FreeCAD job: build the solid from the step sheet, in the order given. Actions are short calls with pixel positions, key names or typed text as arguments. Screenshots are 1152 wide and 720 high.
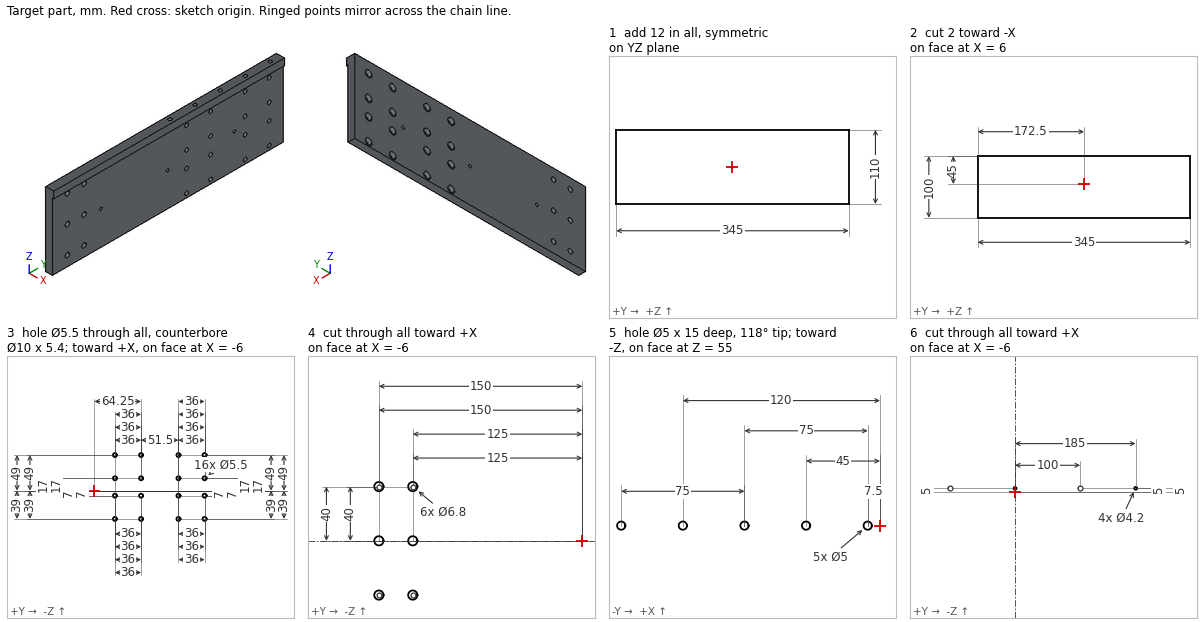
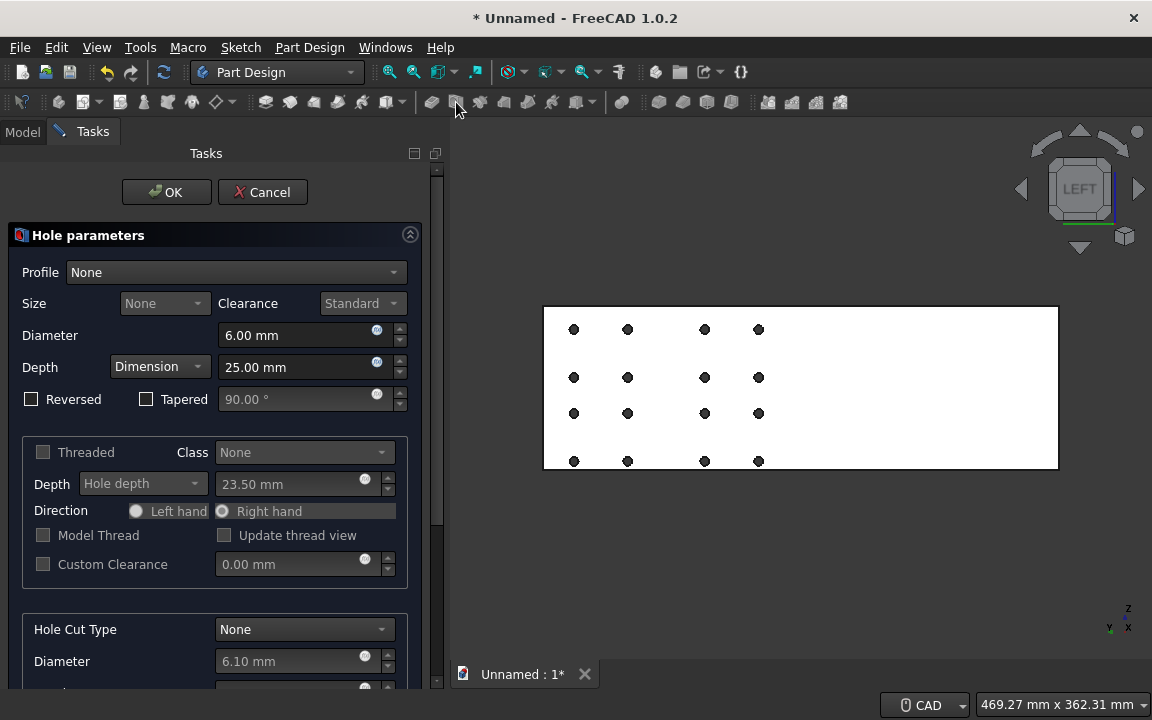
triple_click(305, 335)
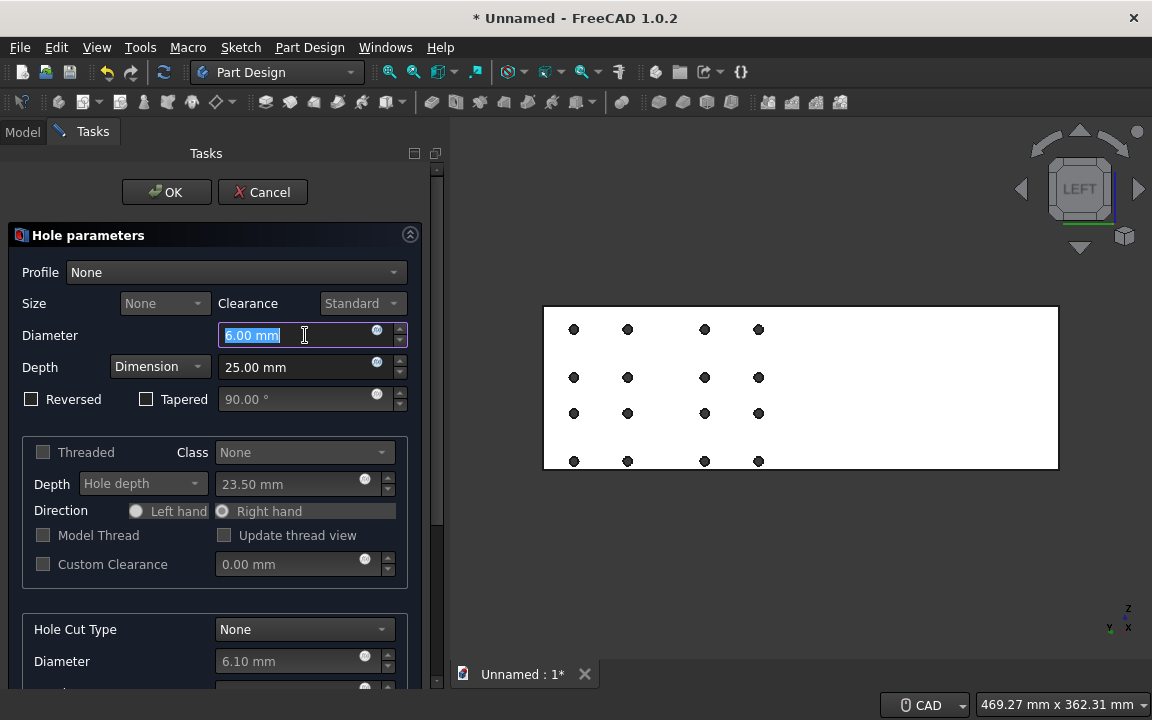
text(5.5)
key(Tab)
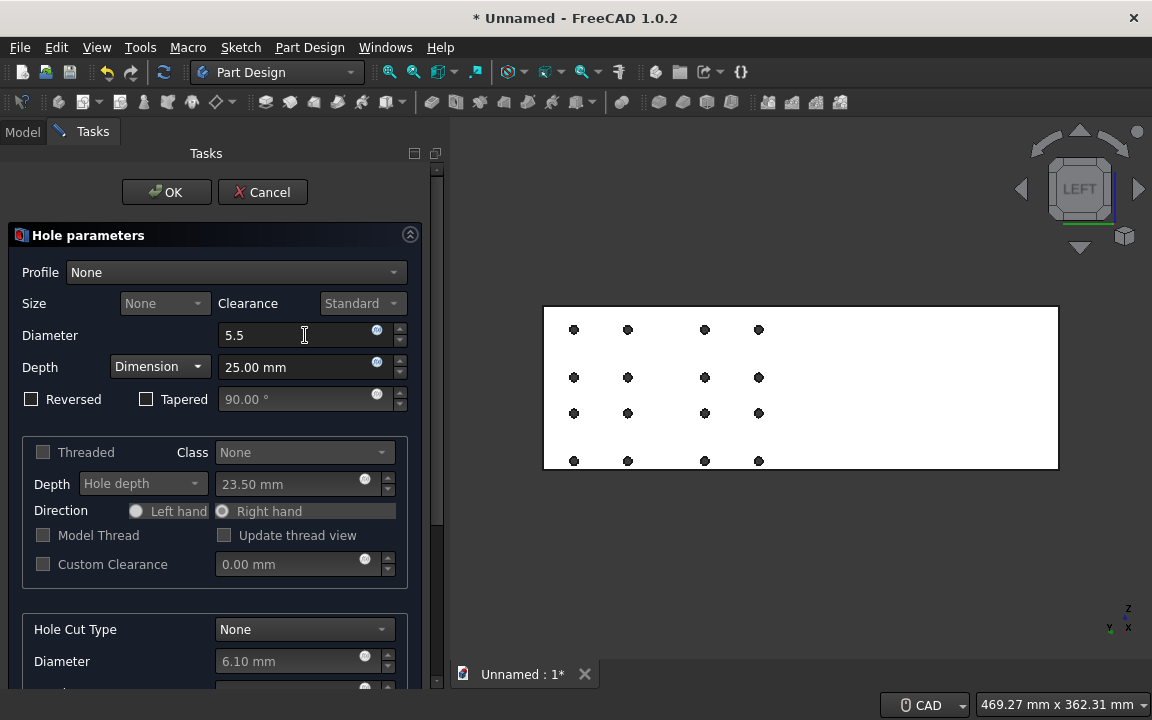
click(161, 366)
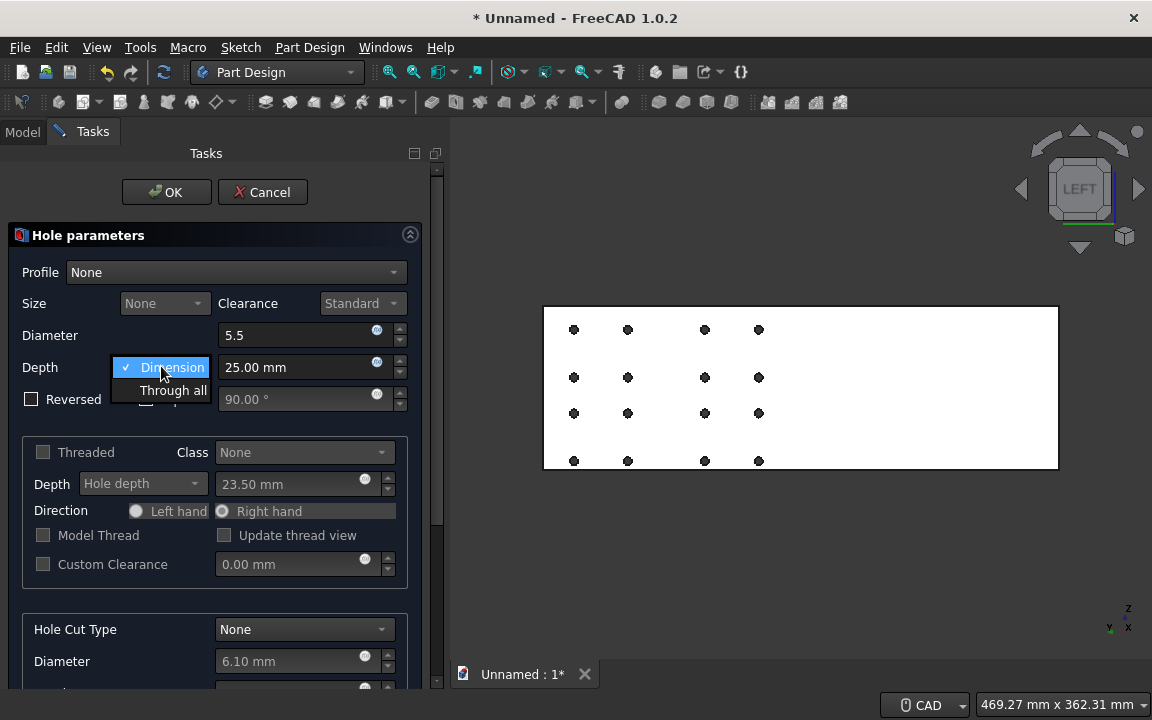
click(160, 390)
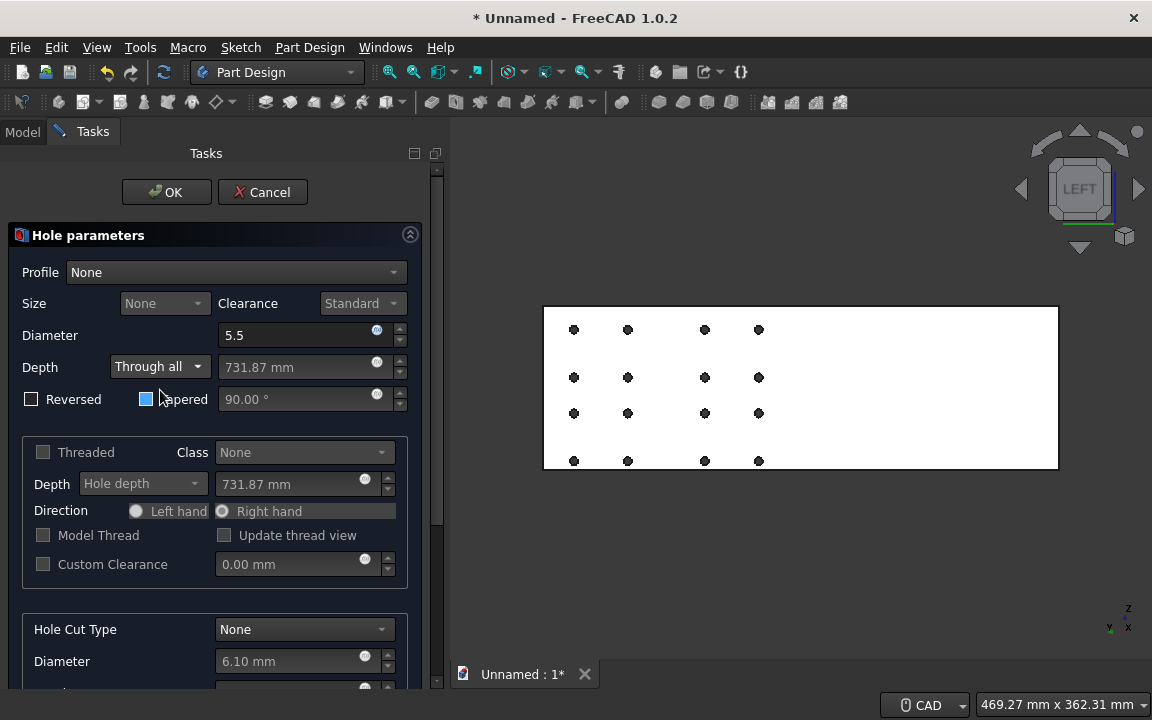
click(306, 630)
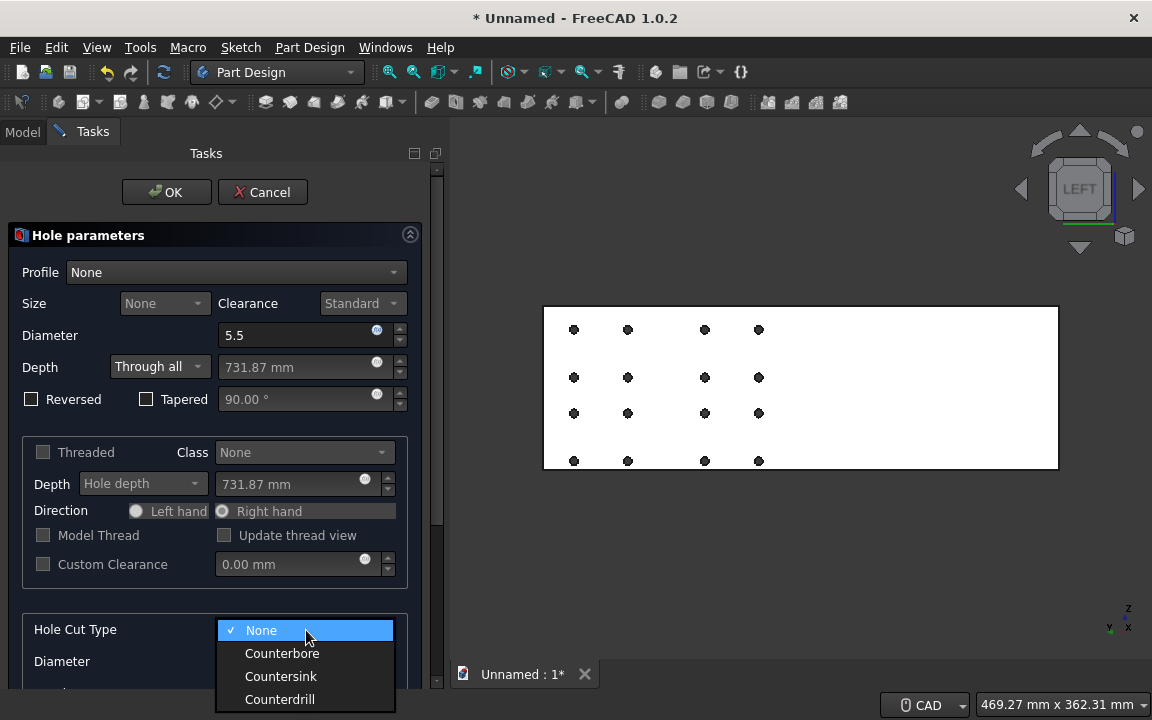
click(304, 654)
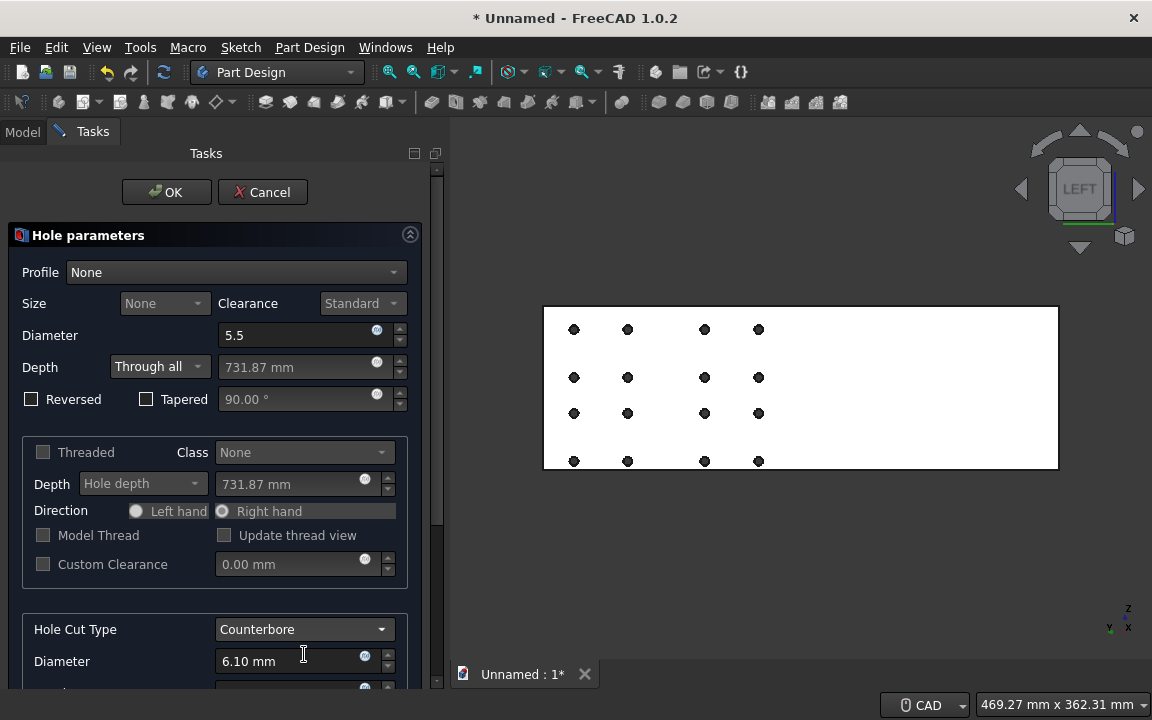
triple_click(298, 661)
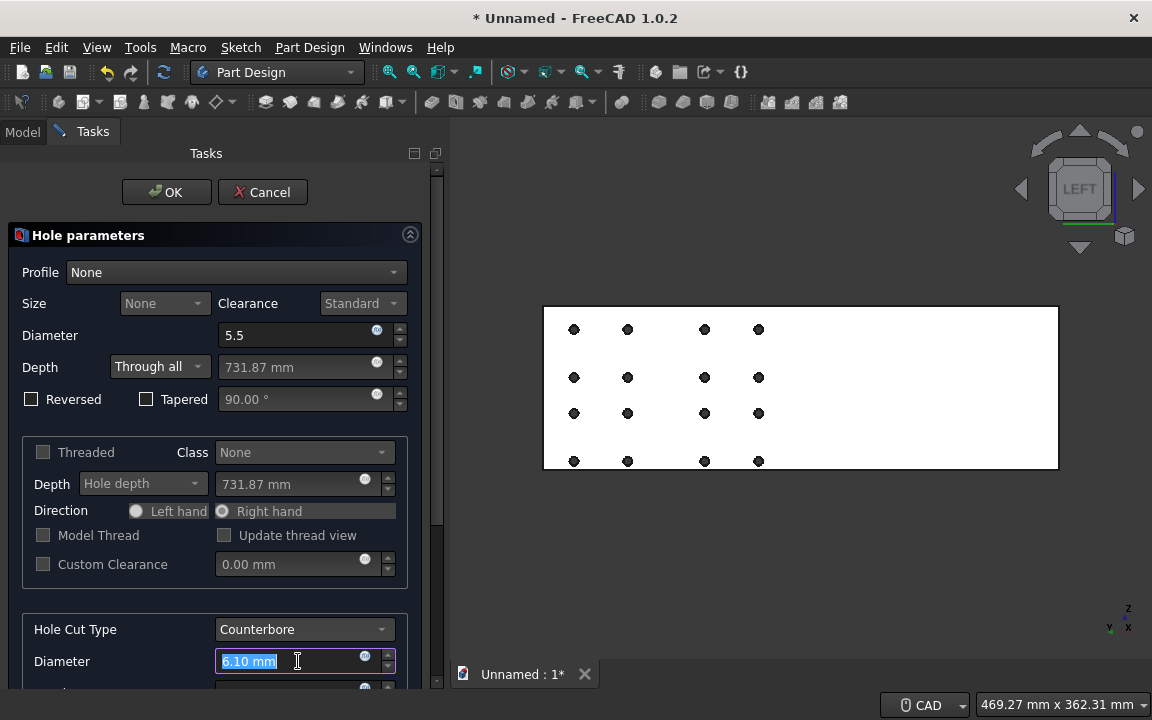
text(10)
key(Tab)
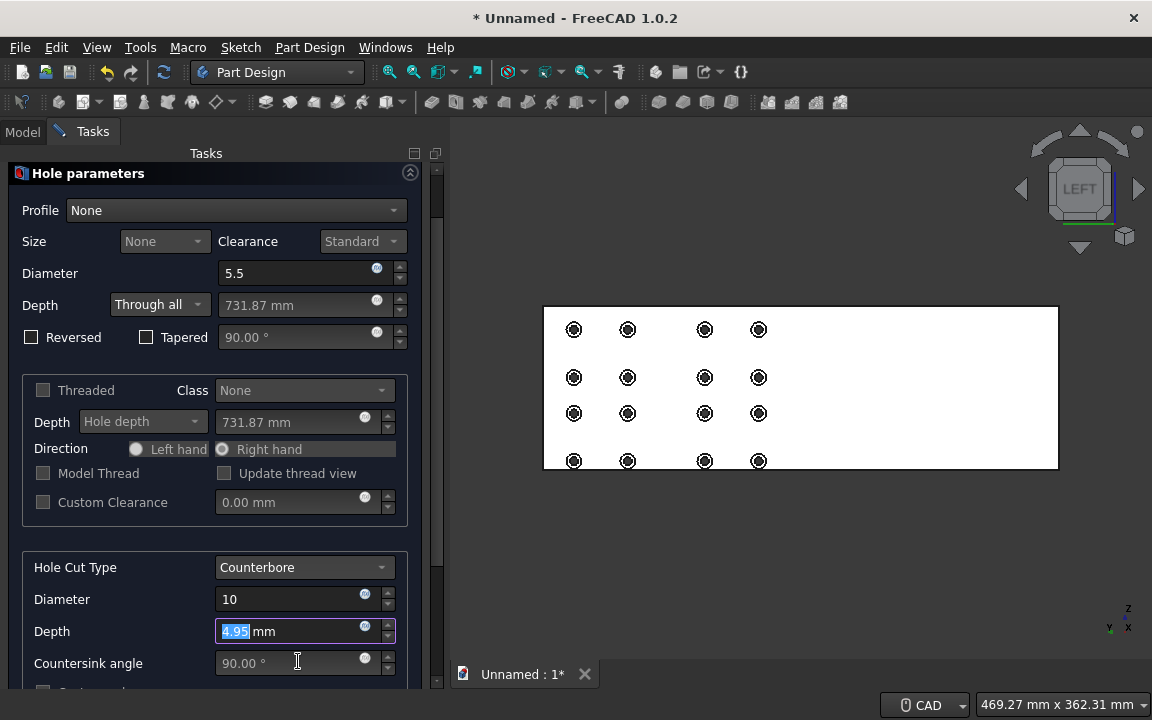
text(5.4)
key(Tab)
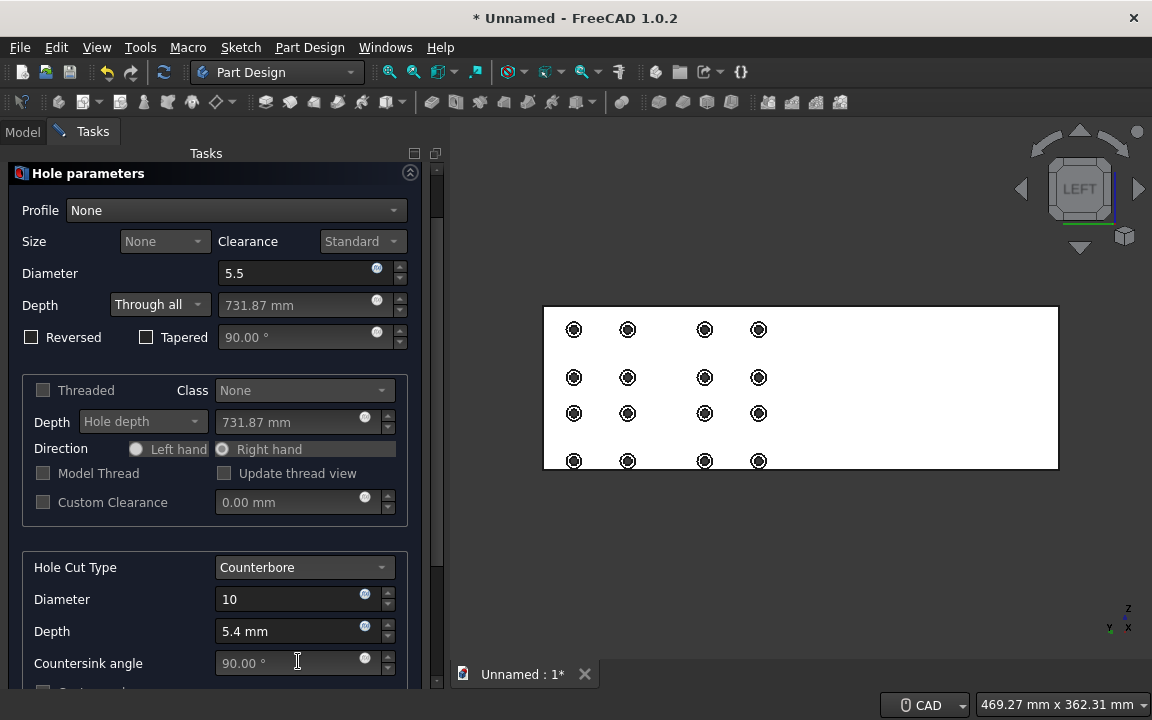
scroll(437, 426, up, 2)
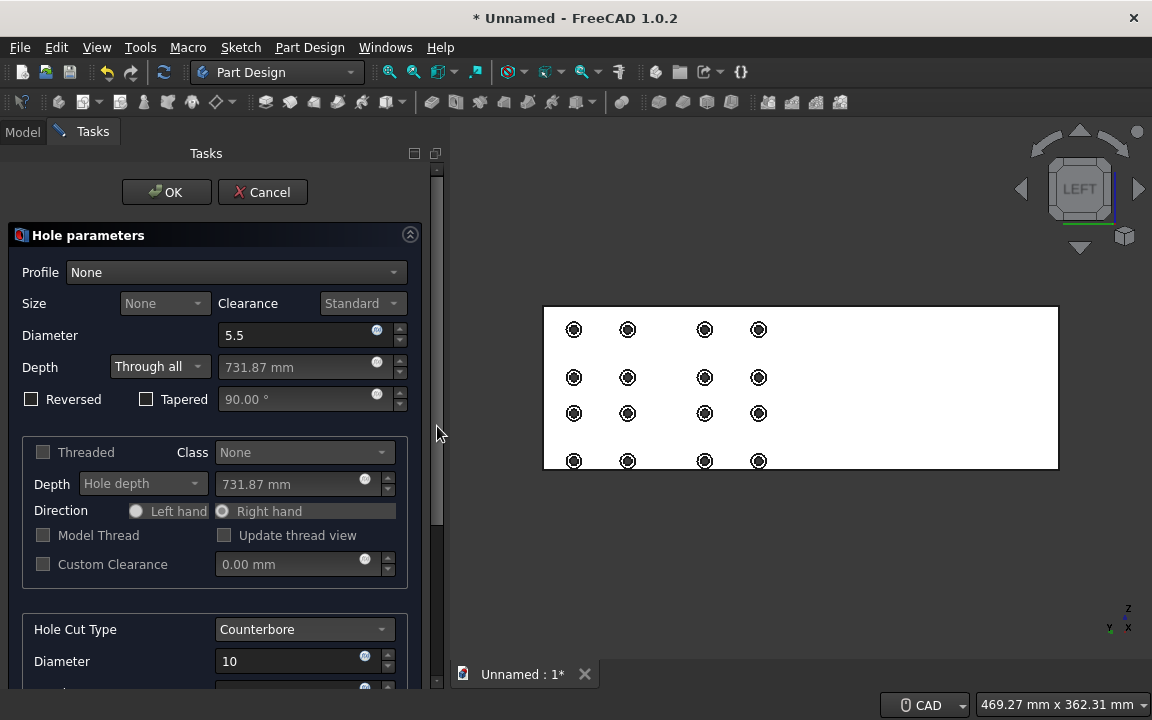
click(167, 192)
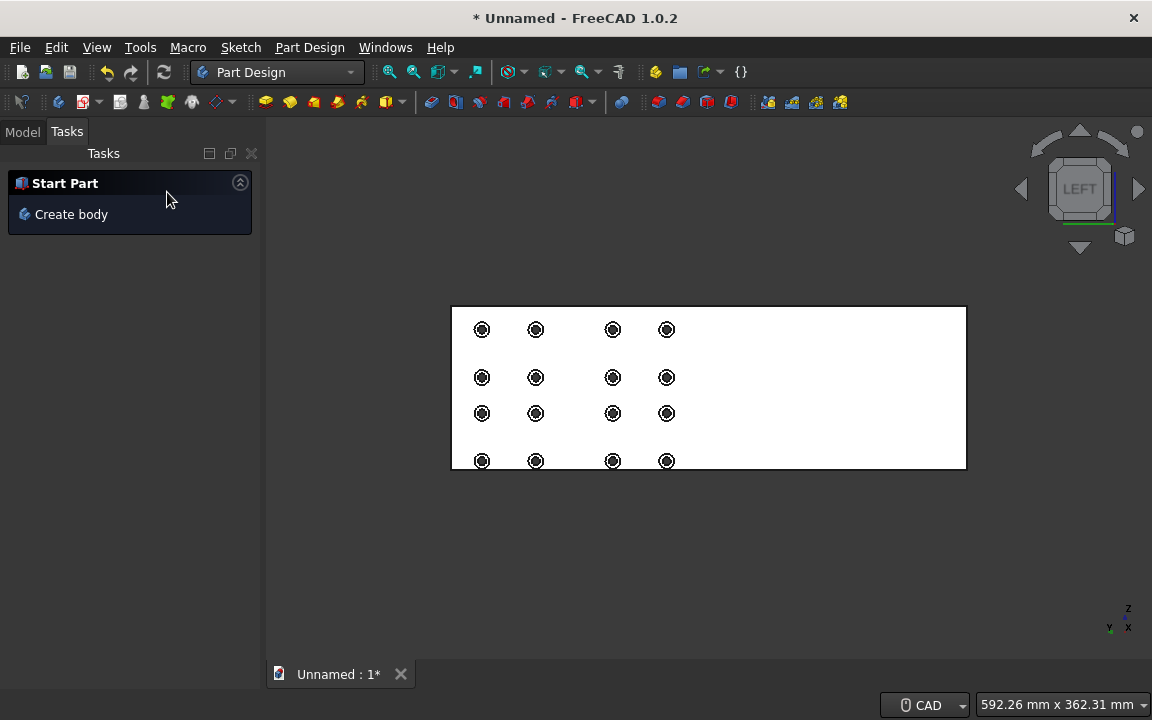
click(783, 387)